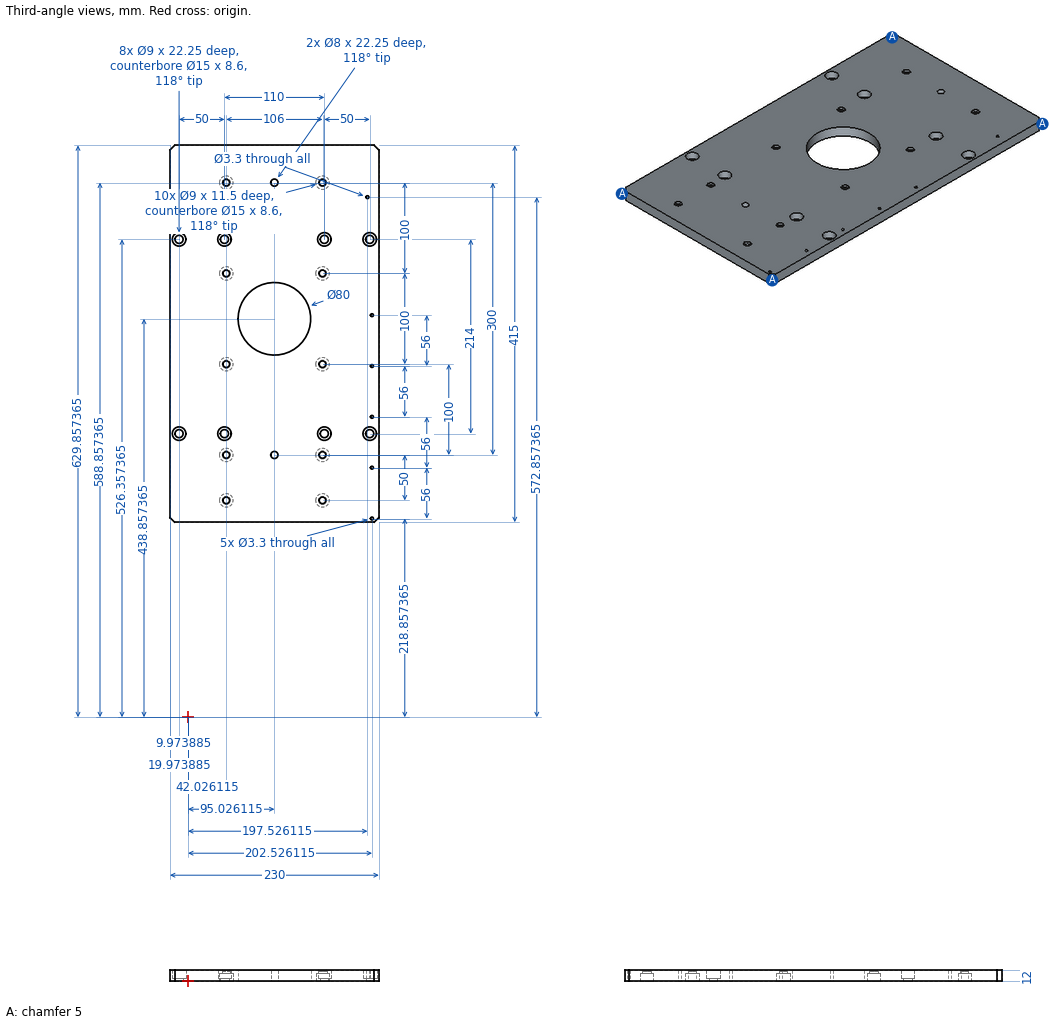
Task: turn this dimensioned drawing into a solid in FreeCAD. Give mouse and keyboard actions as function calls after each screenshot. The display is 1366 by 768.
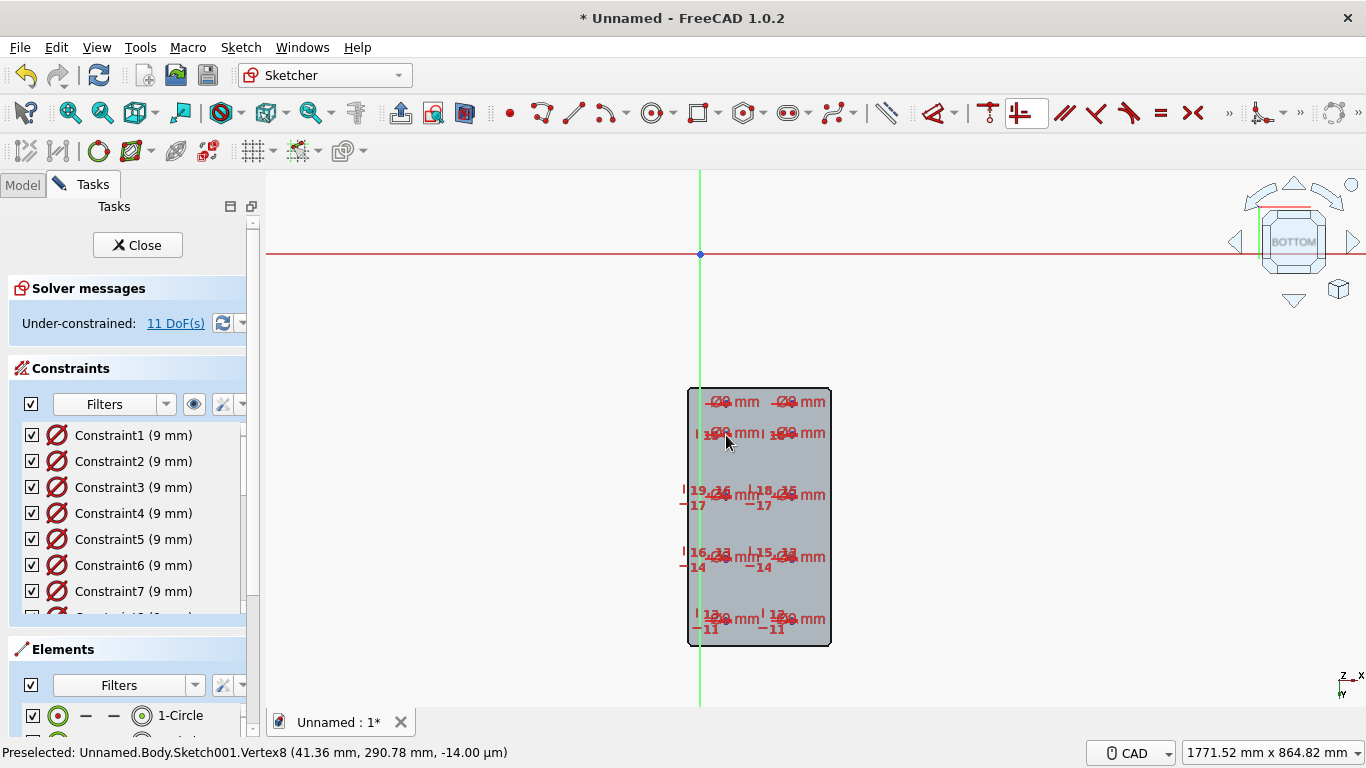
click(792, 435)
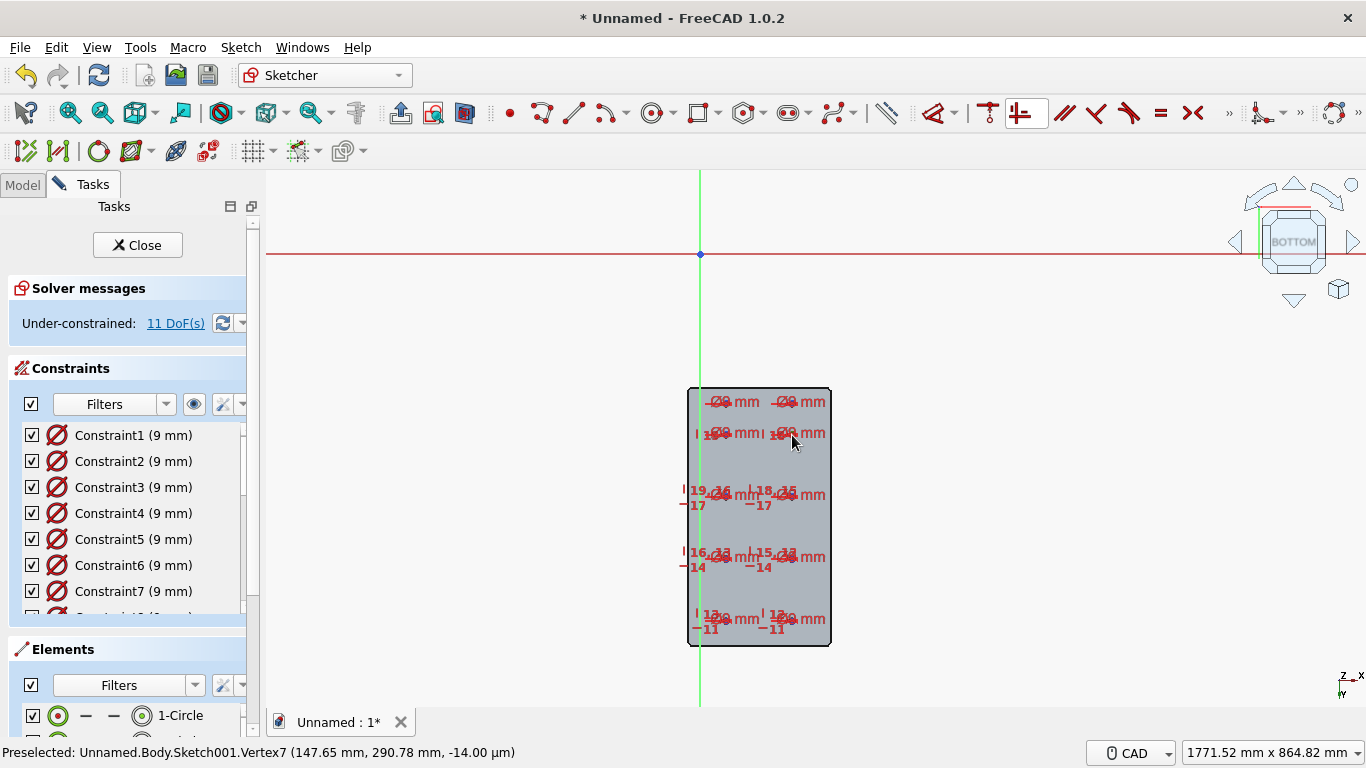
click(726, 435)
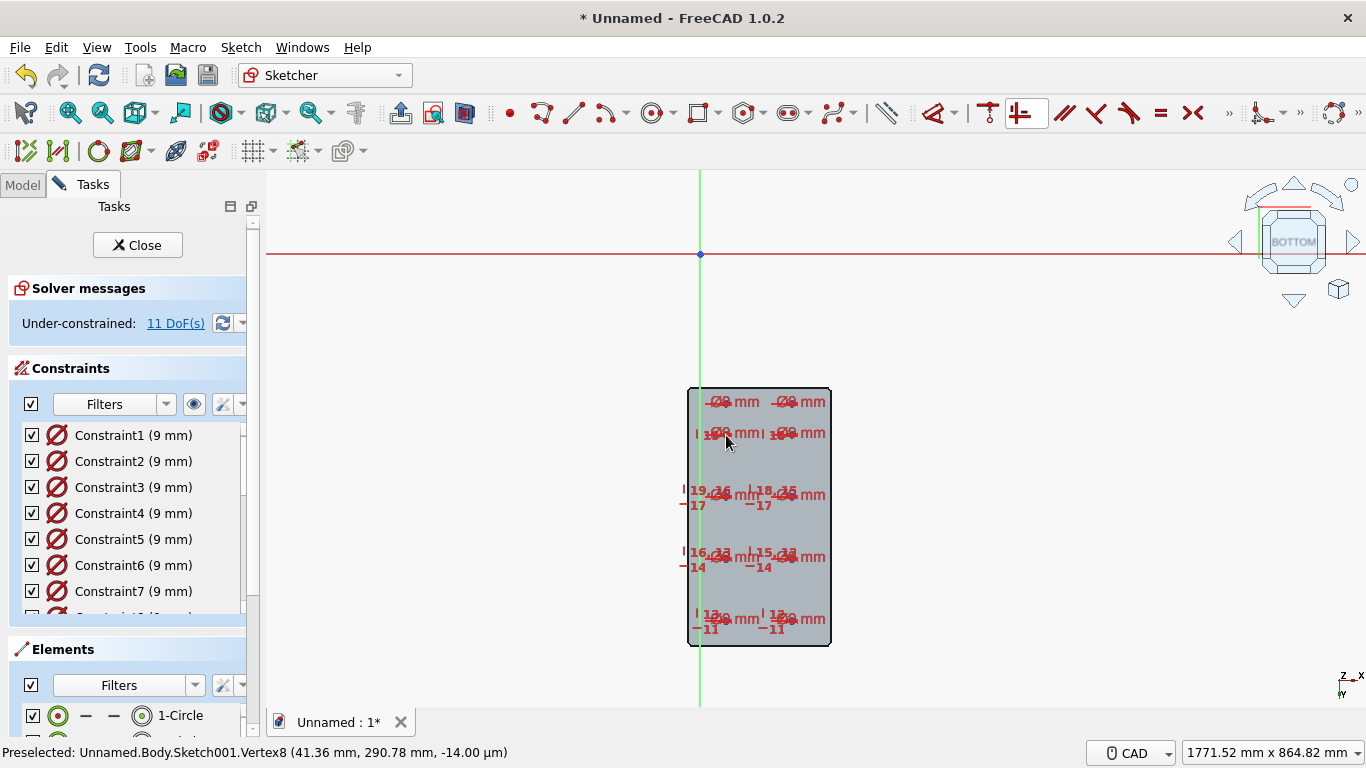
click(1042, 114)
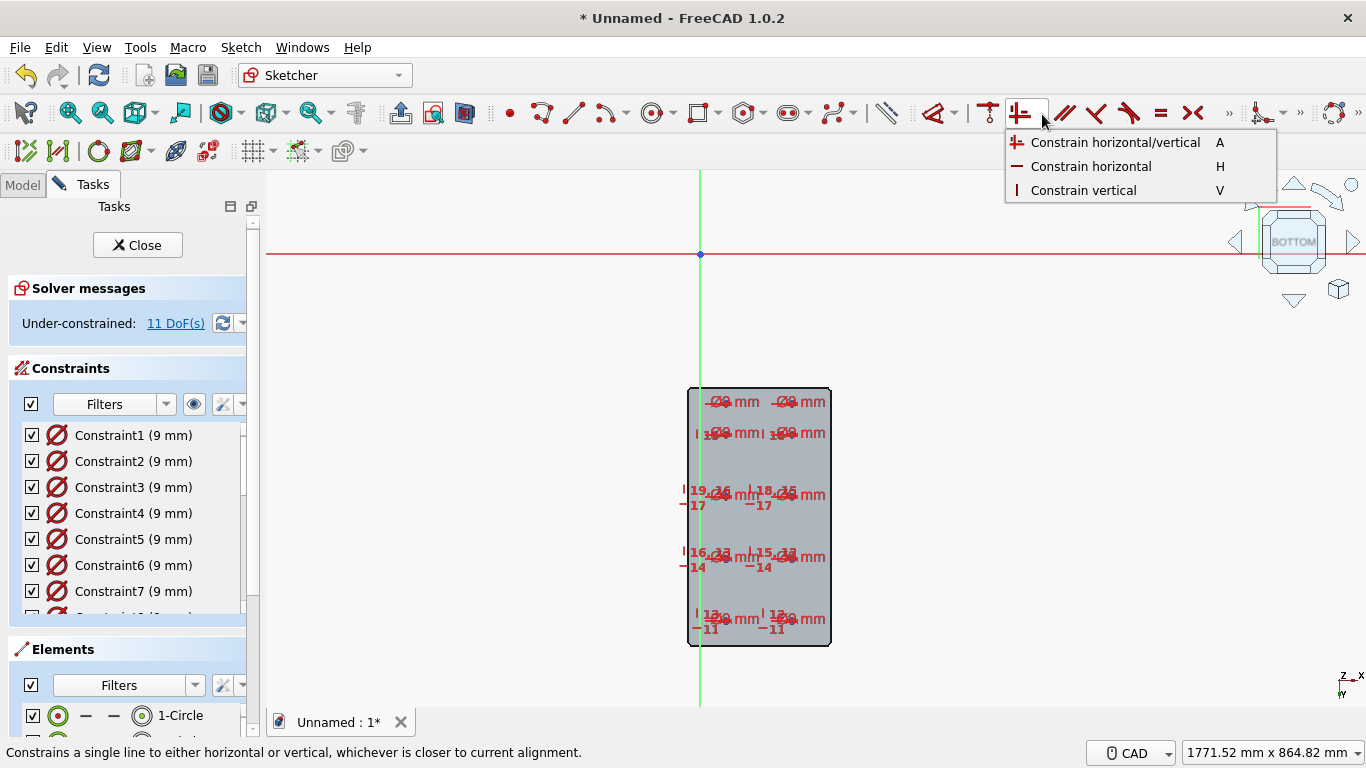
click(1141, 166)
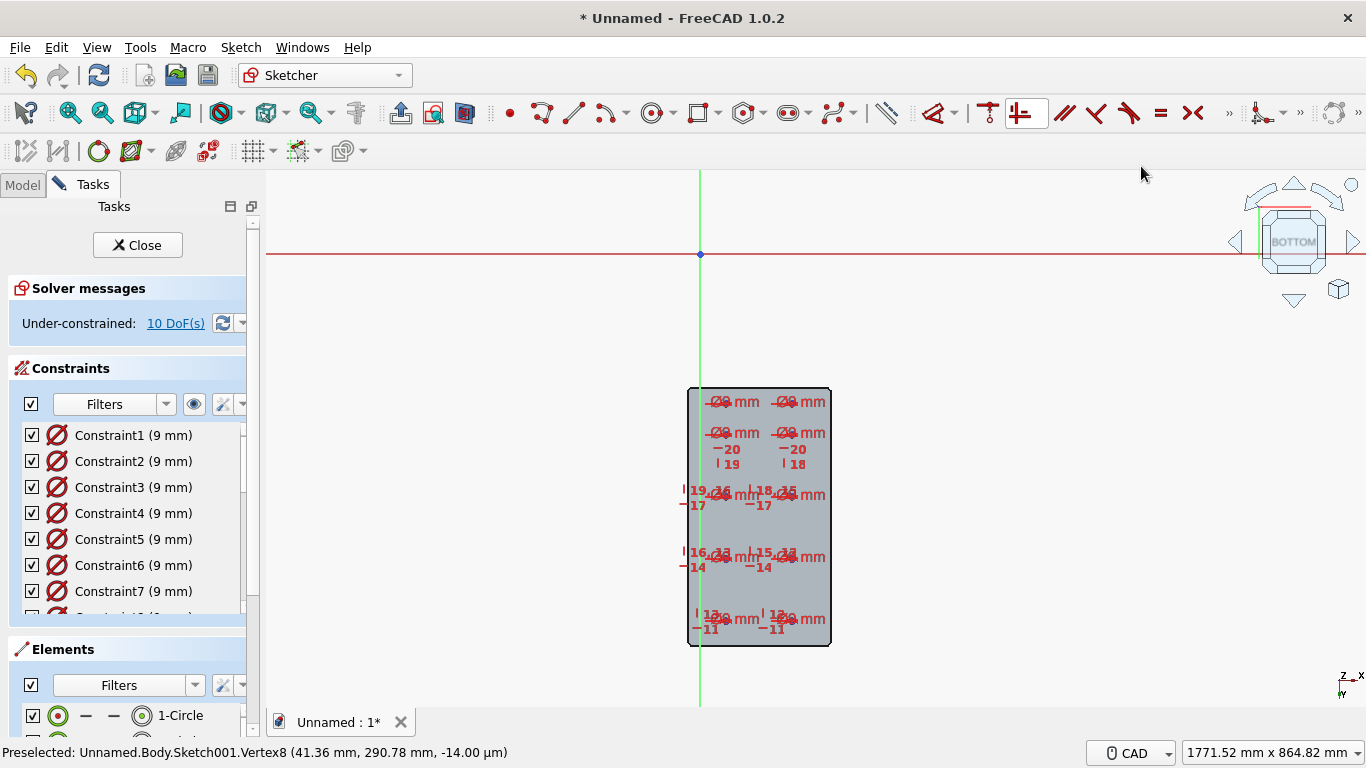
click(792, 435)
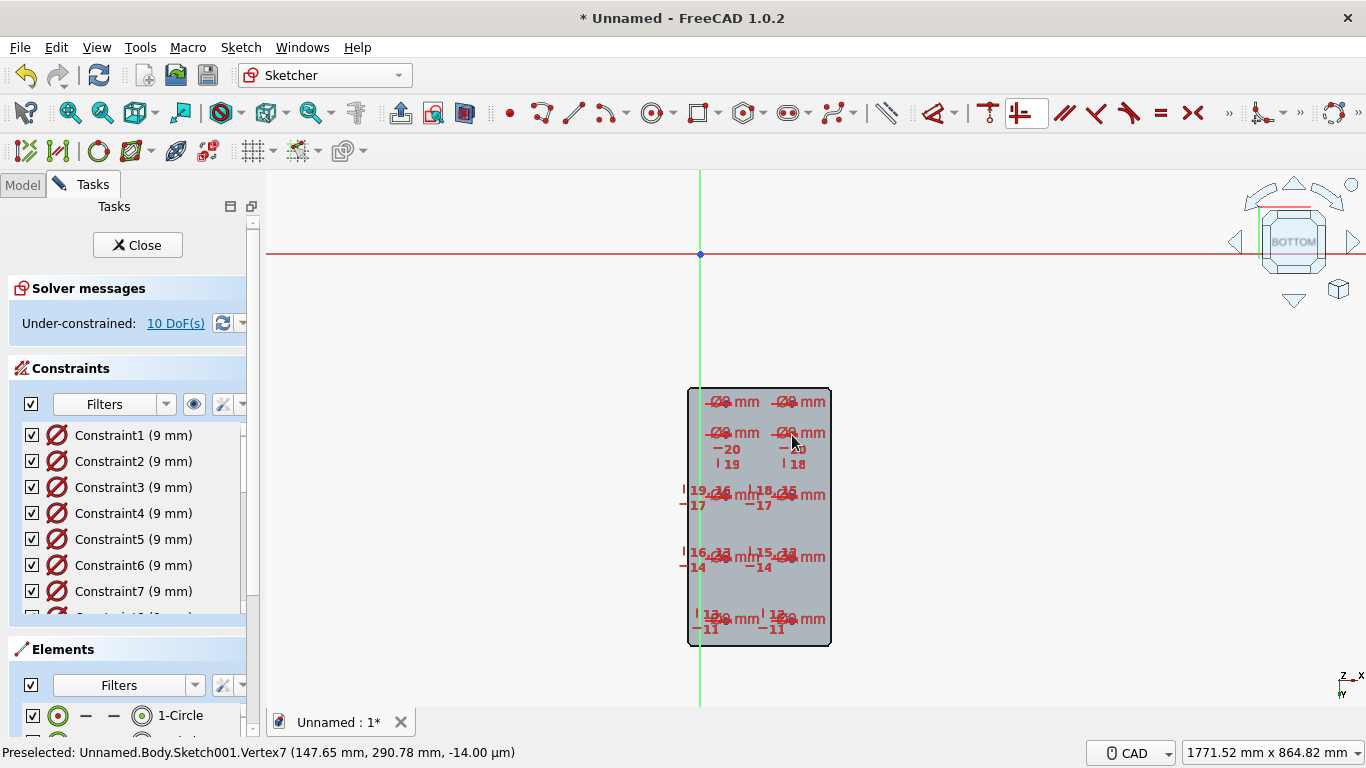
click(792, 404)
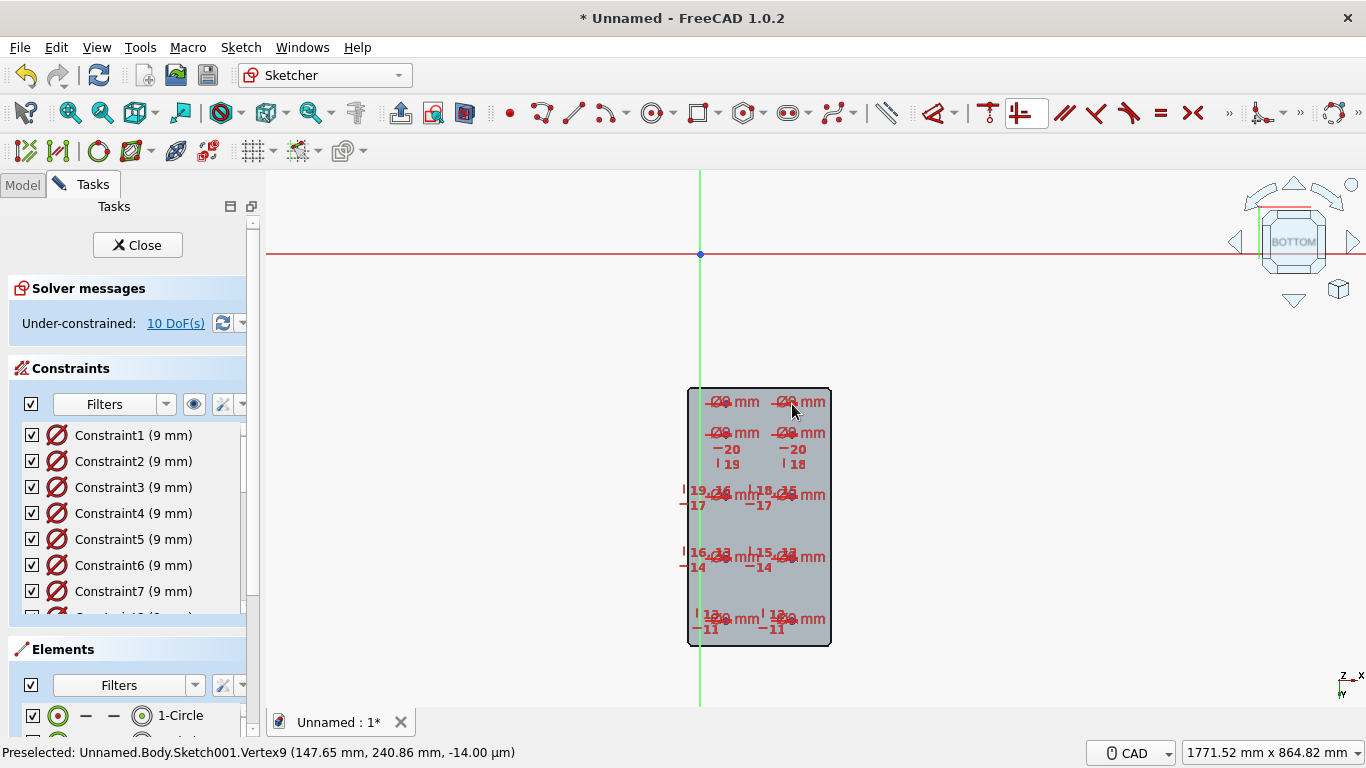
key(v)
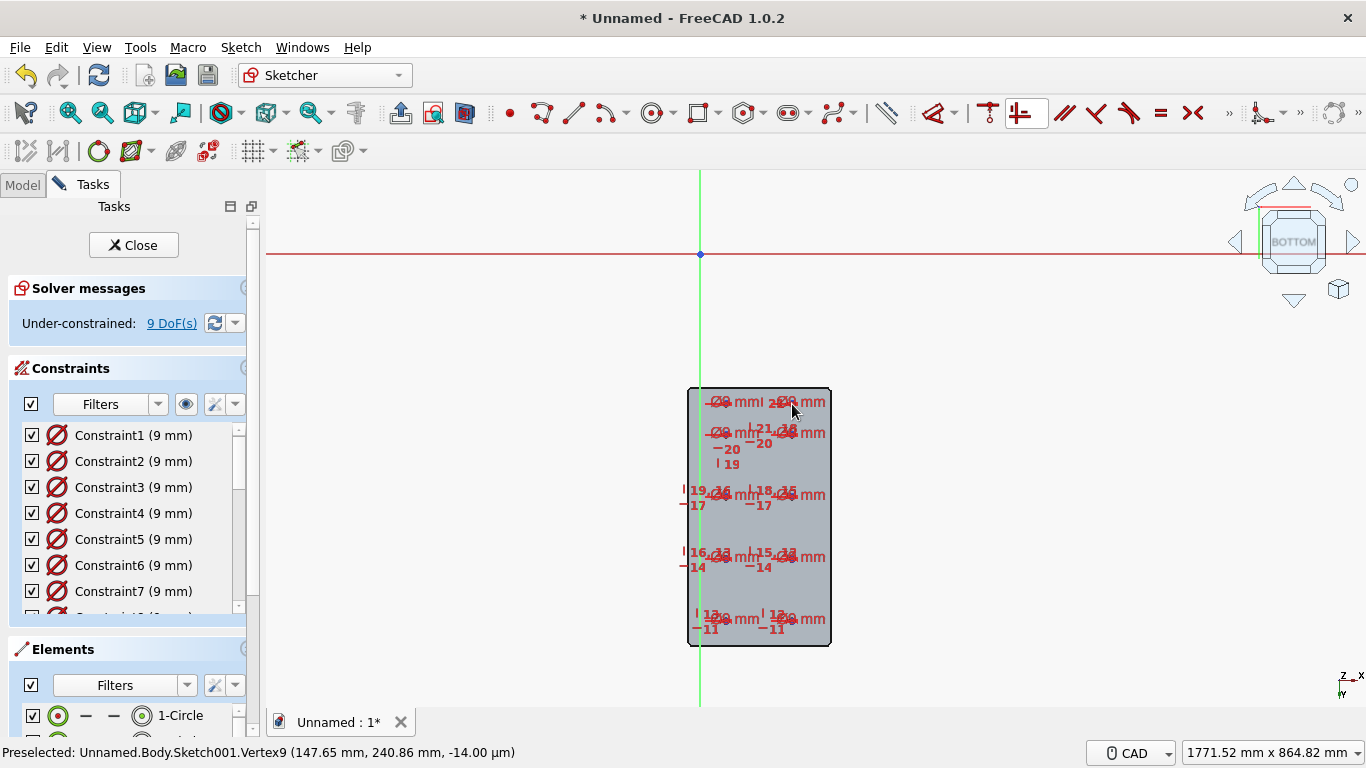
click(726, 435)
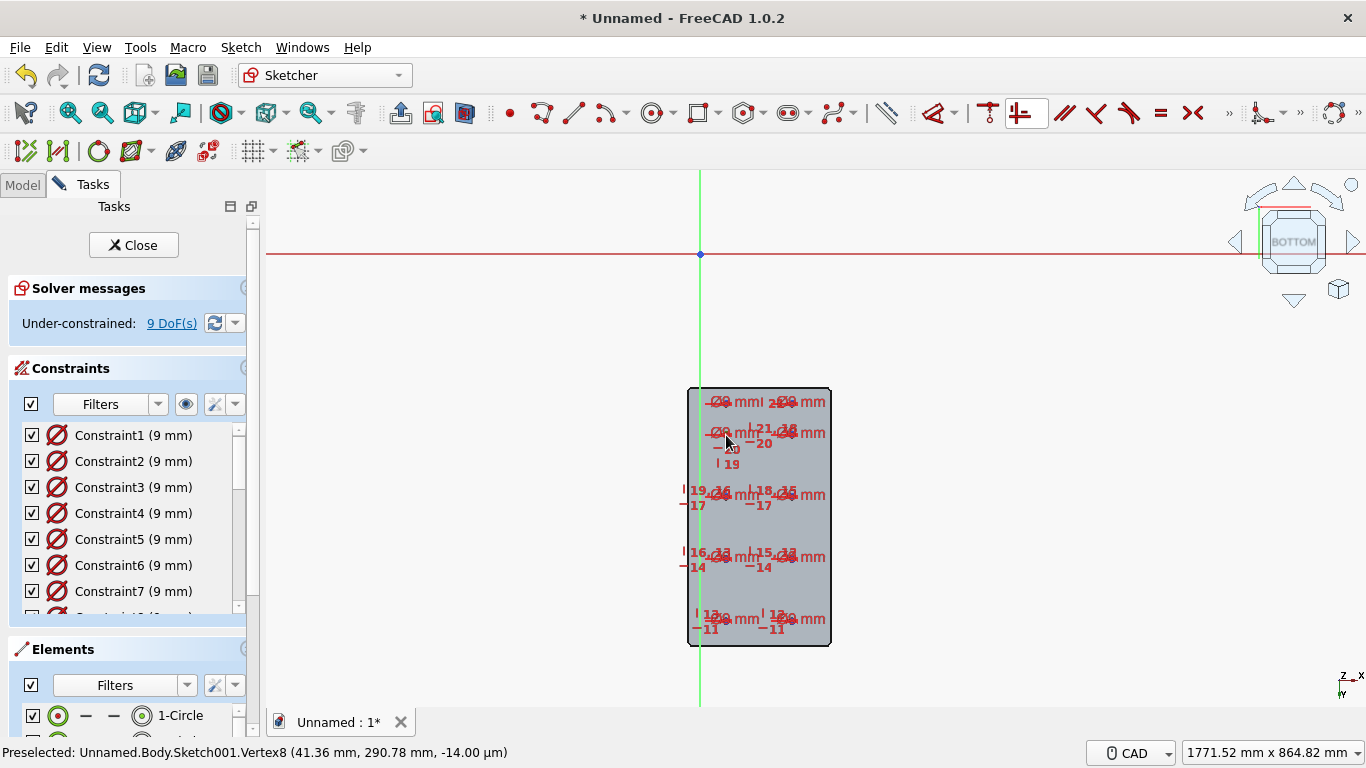
click(726, 404)